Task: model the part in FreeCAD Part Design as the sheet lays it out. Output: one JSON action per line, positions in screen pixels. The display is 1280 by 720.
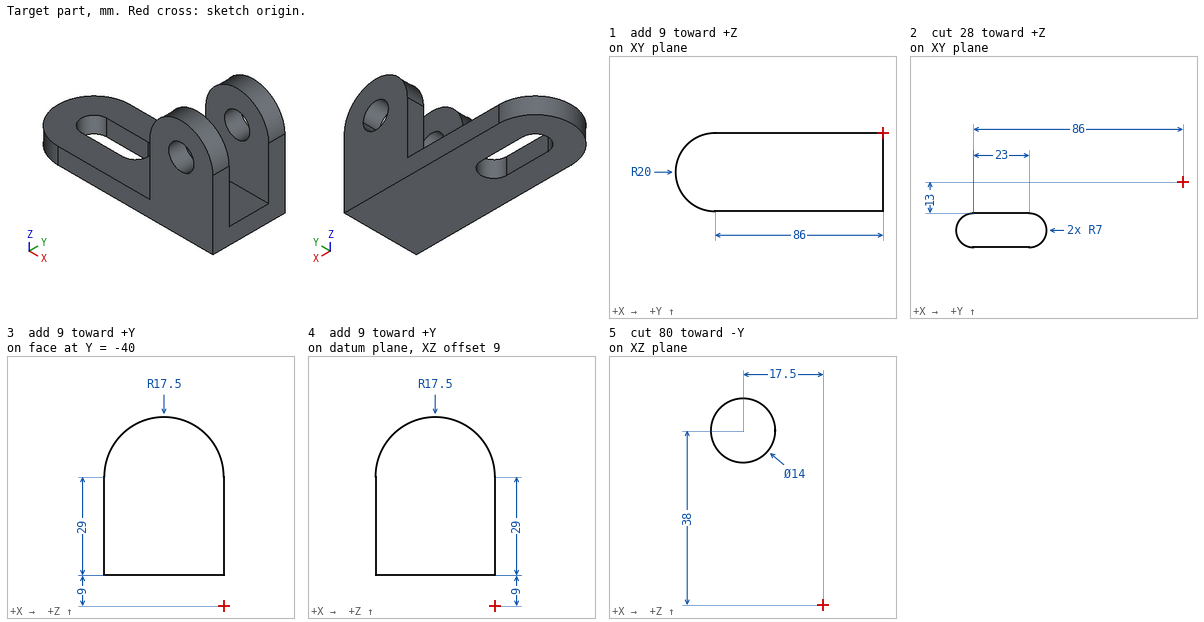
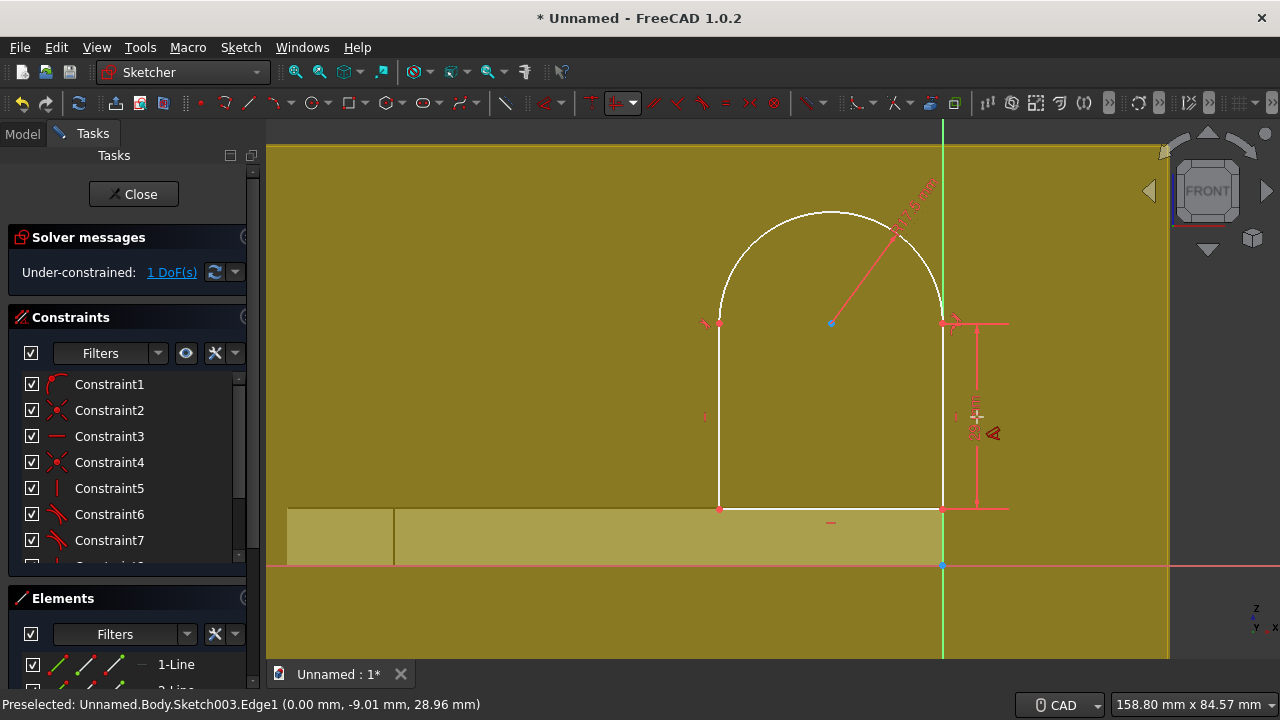
{"action": "left_click", "coordinate": [943, 509]}
{"action": "left_click", "coordinate": [977, 537]}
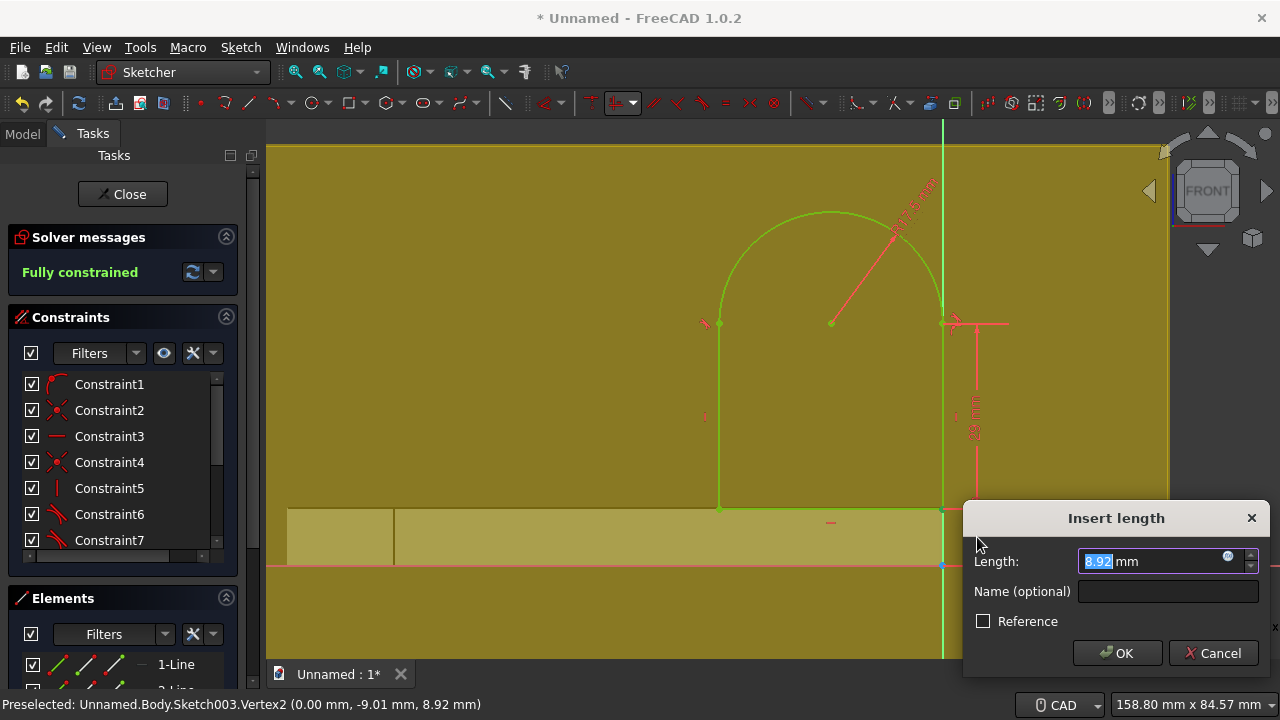
{"action": "type", "text": "9"}
{"action": "key", "text": "Return"}
{"action": "key", "text": "Escape"}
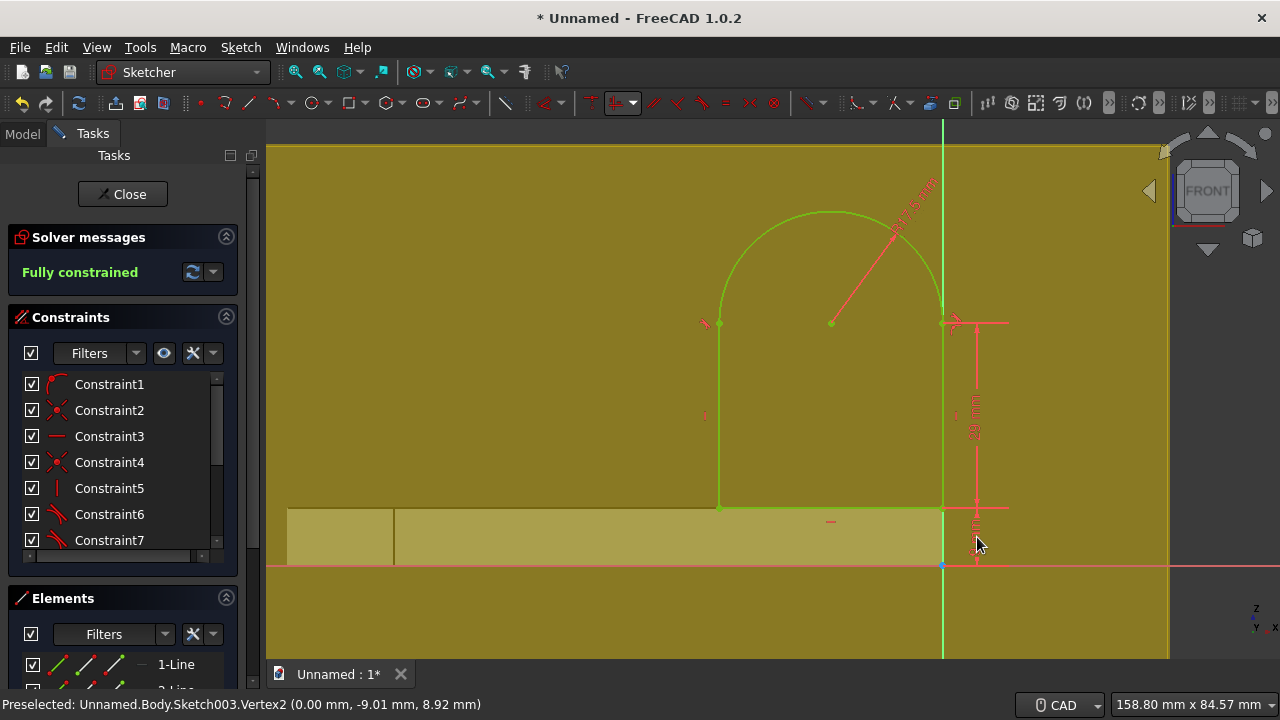
{"action": "left_click", "coordinate": [123, 194]}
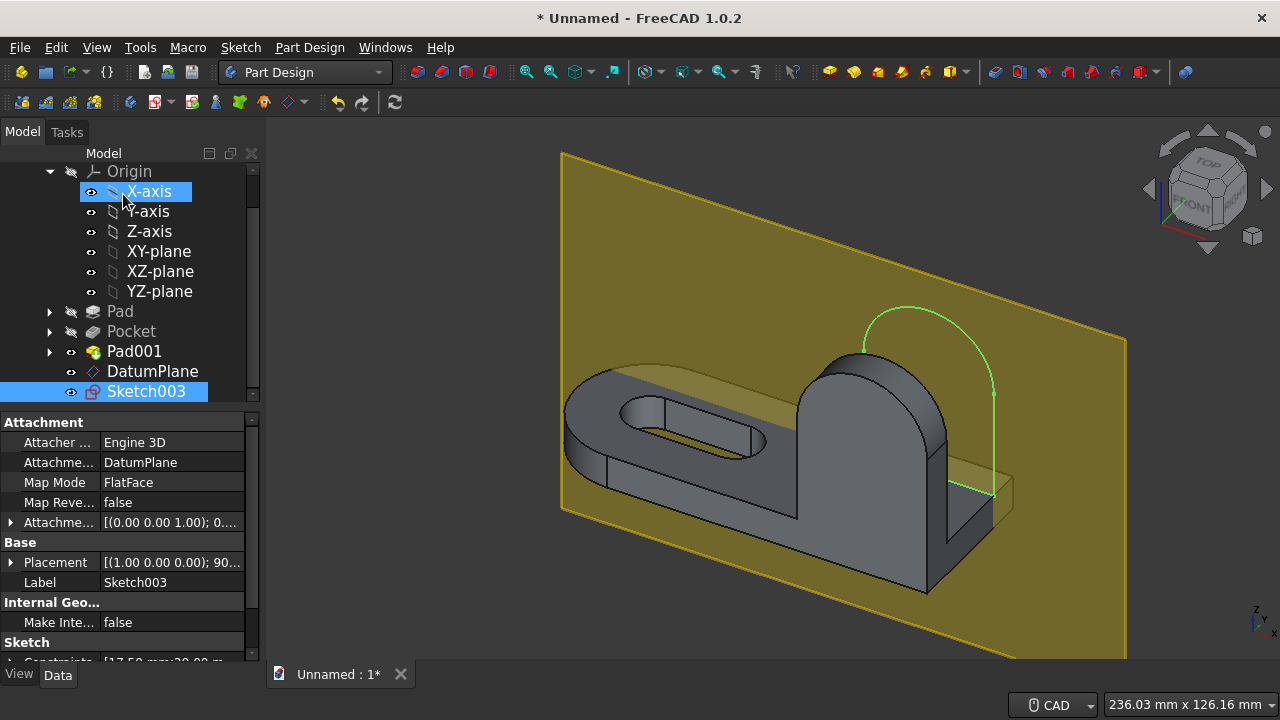
{"action": "left_click", "coordinate": [830, 72]}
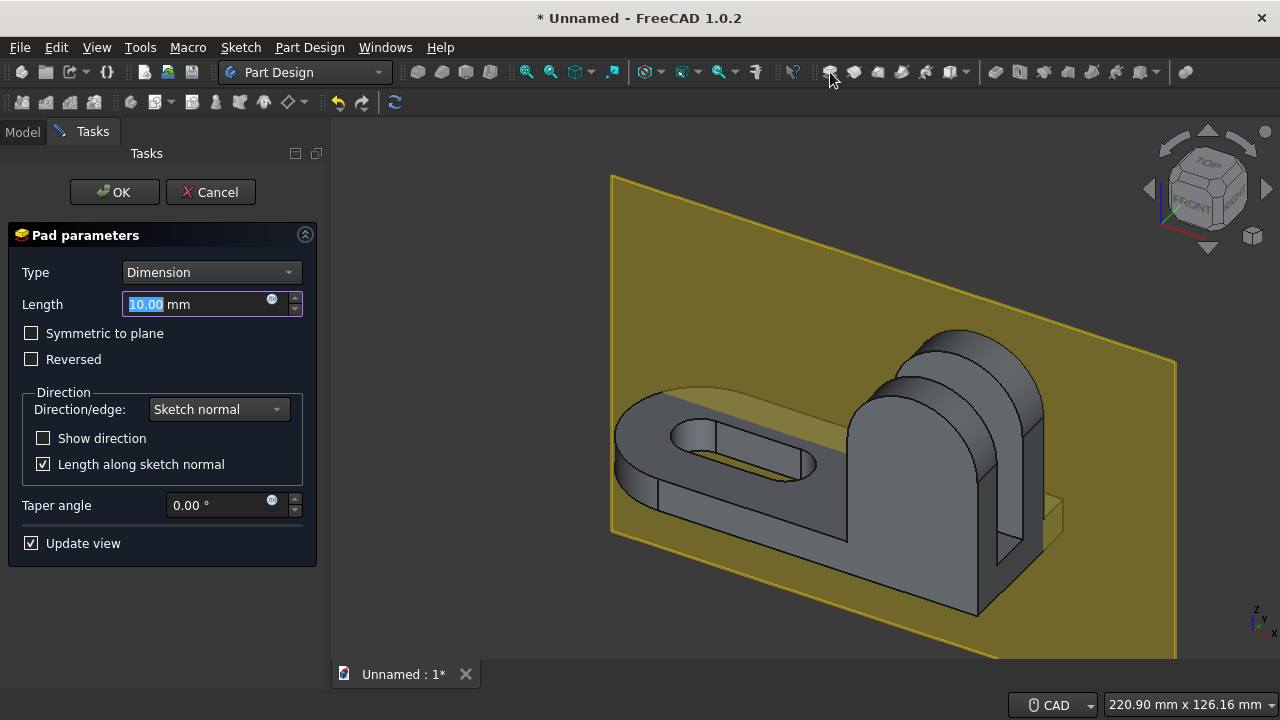
{"action": "type", "text": "9"}
{"action": "key", "text": "Tab"}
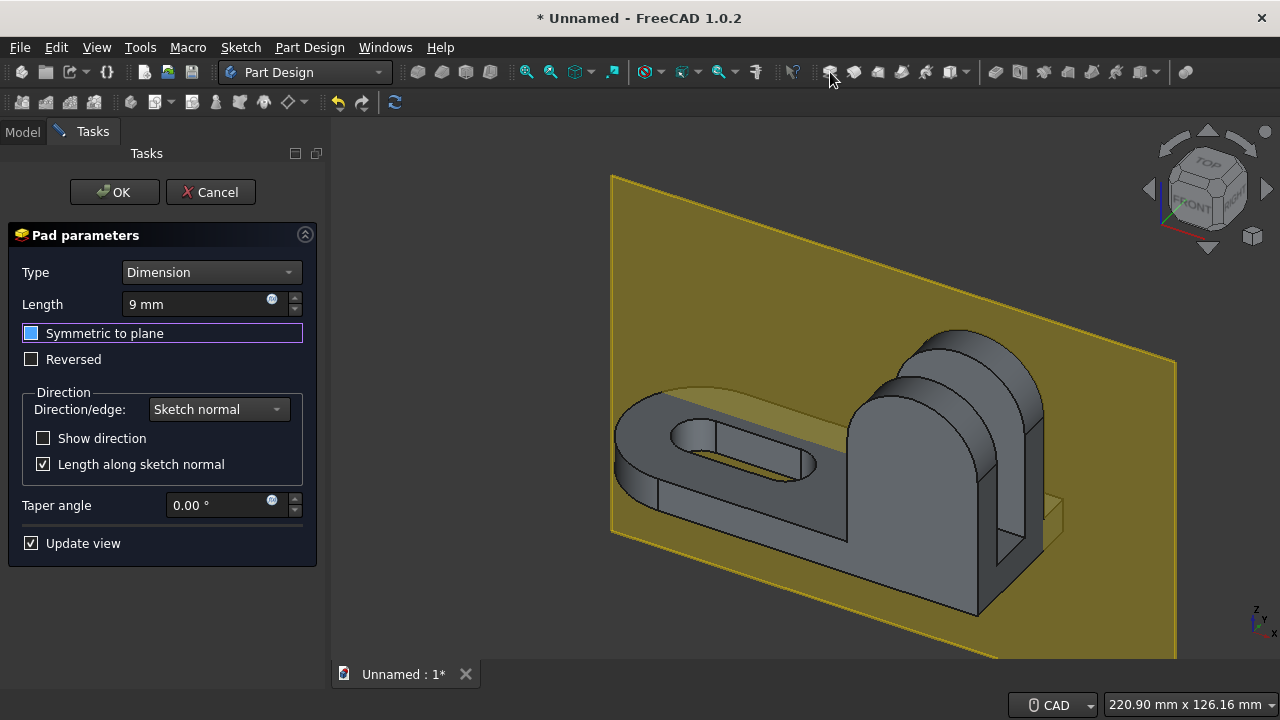
{"action": "left_click", "coordinate": [30, 359]}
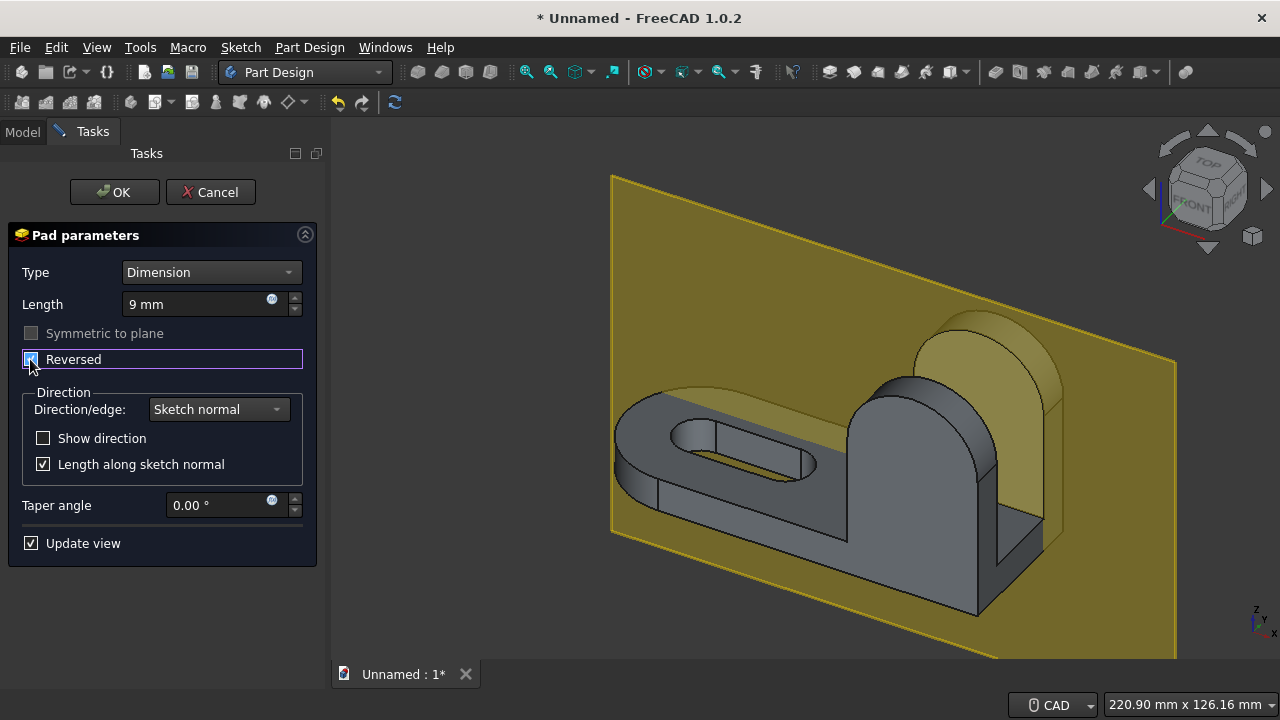
{"action": "left_click", "coordinate": [115, 192]}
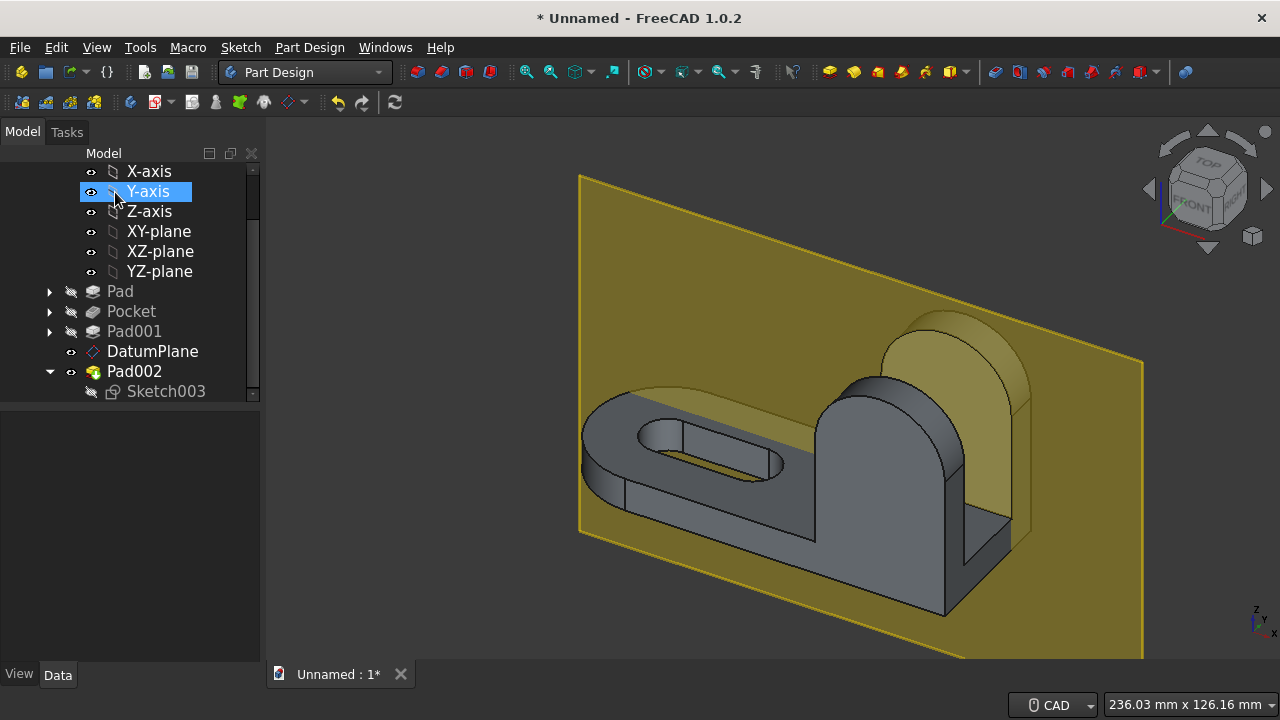
{"action": "left_click", "coordinate": [116, 352]}
{"action": "key", "text": "space"}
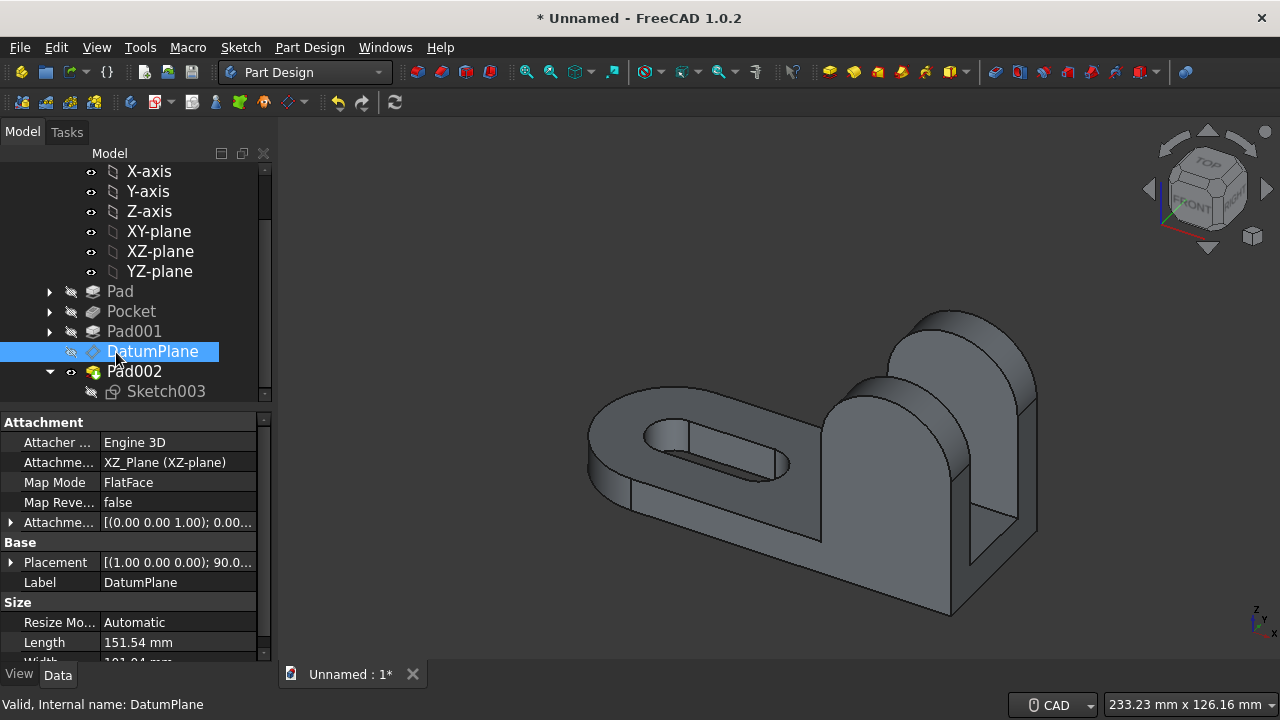
{"action": "left_click", "coordinate": [318, 619]}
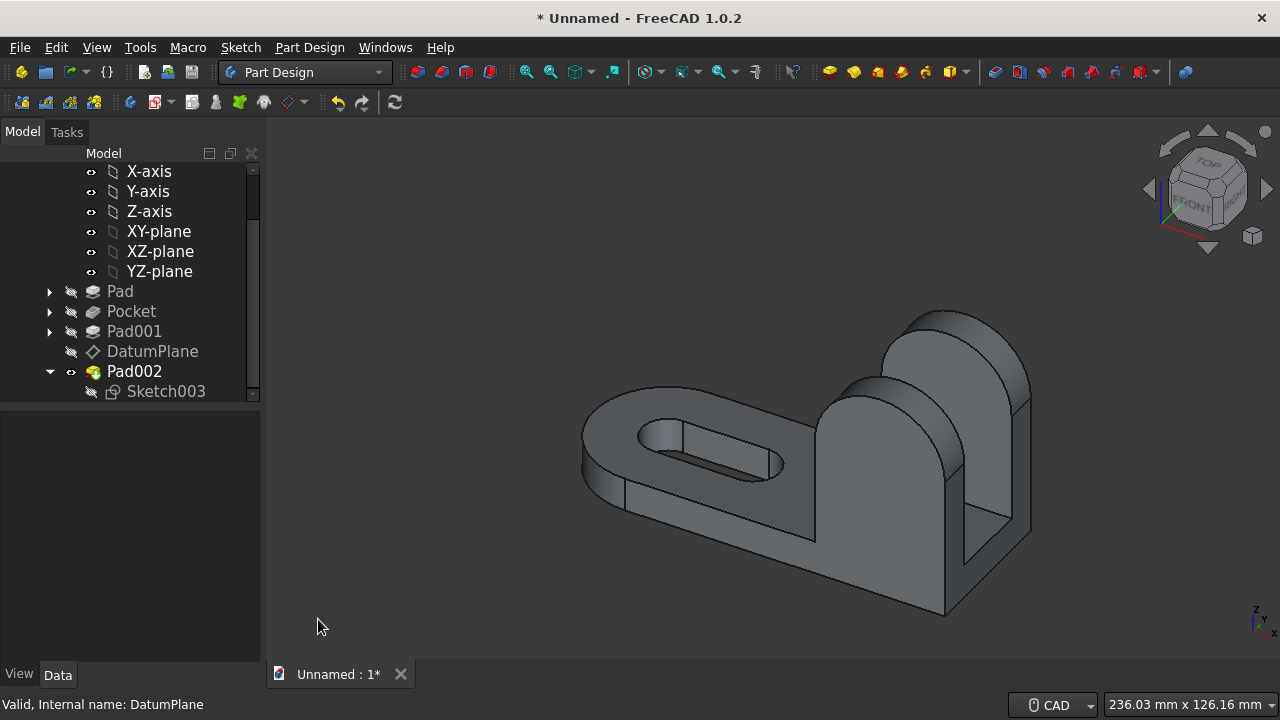
{"action": "left_click", "coordinate": [156, 102]}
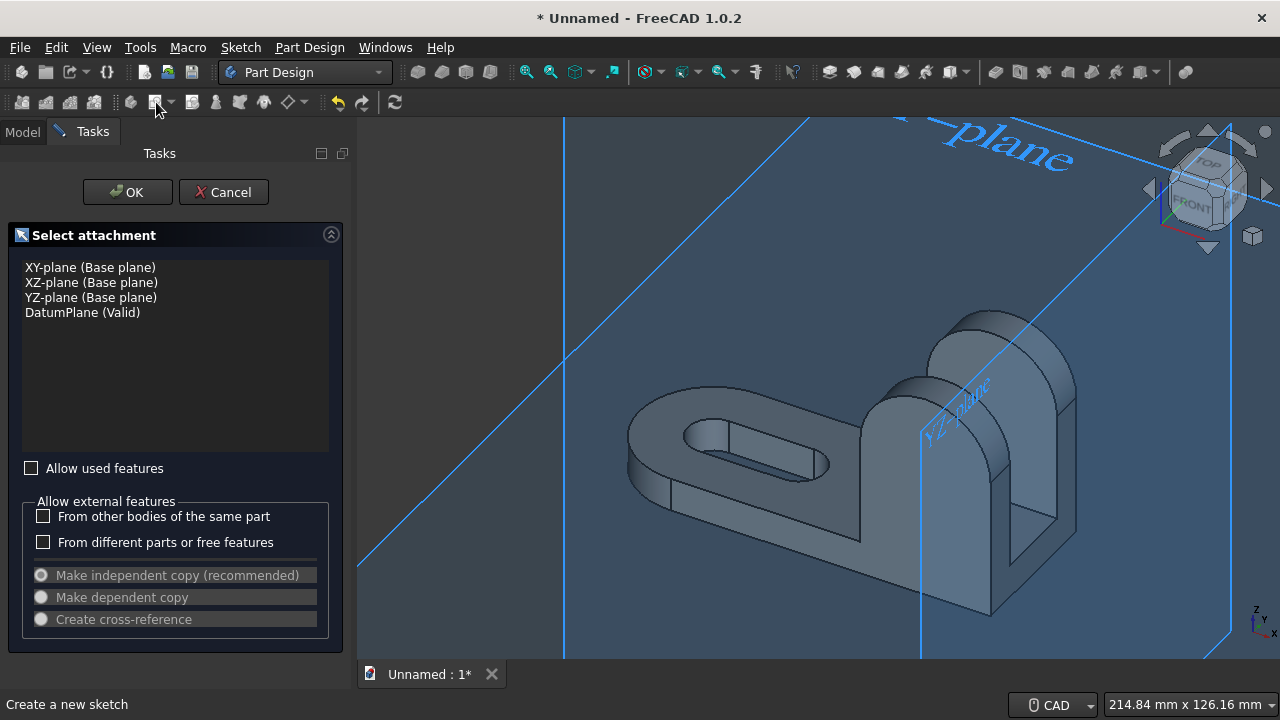
{"action": "left_click", "coordinate": [82, 282]}